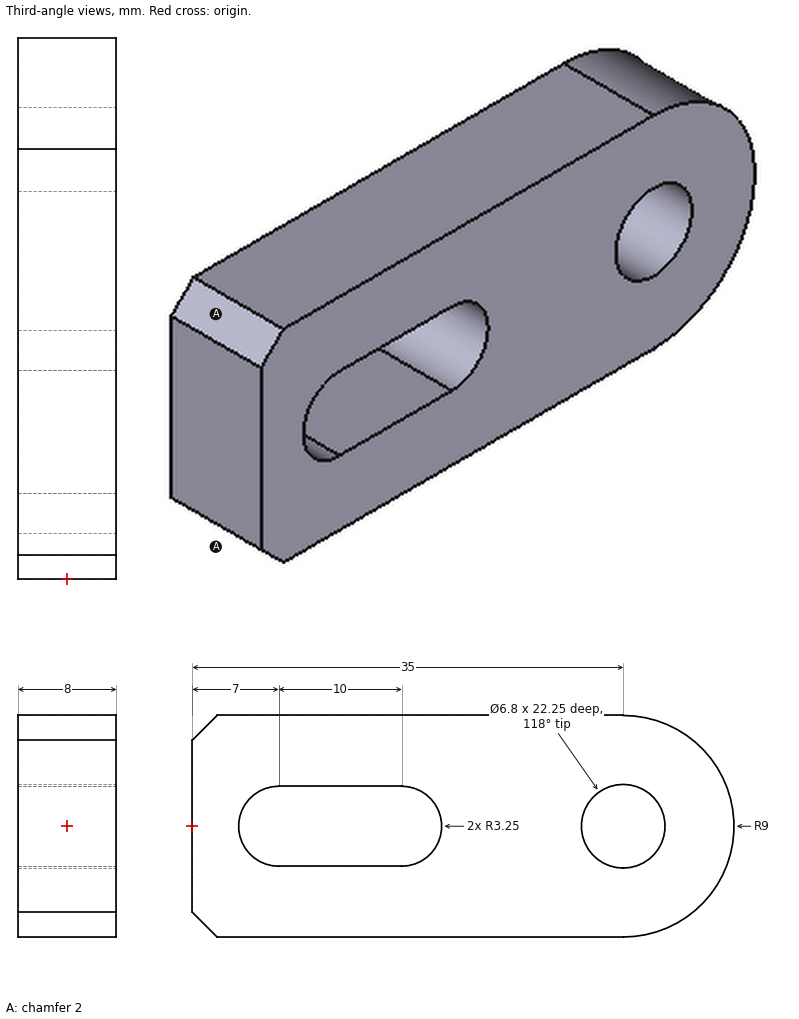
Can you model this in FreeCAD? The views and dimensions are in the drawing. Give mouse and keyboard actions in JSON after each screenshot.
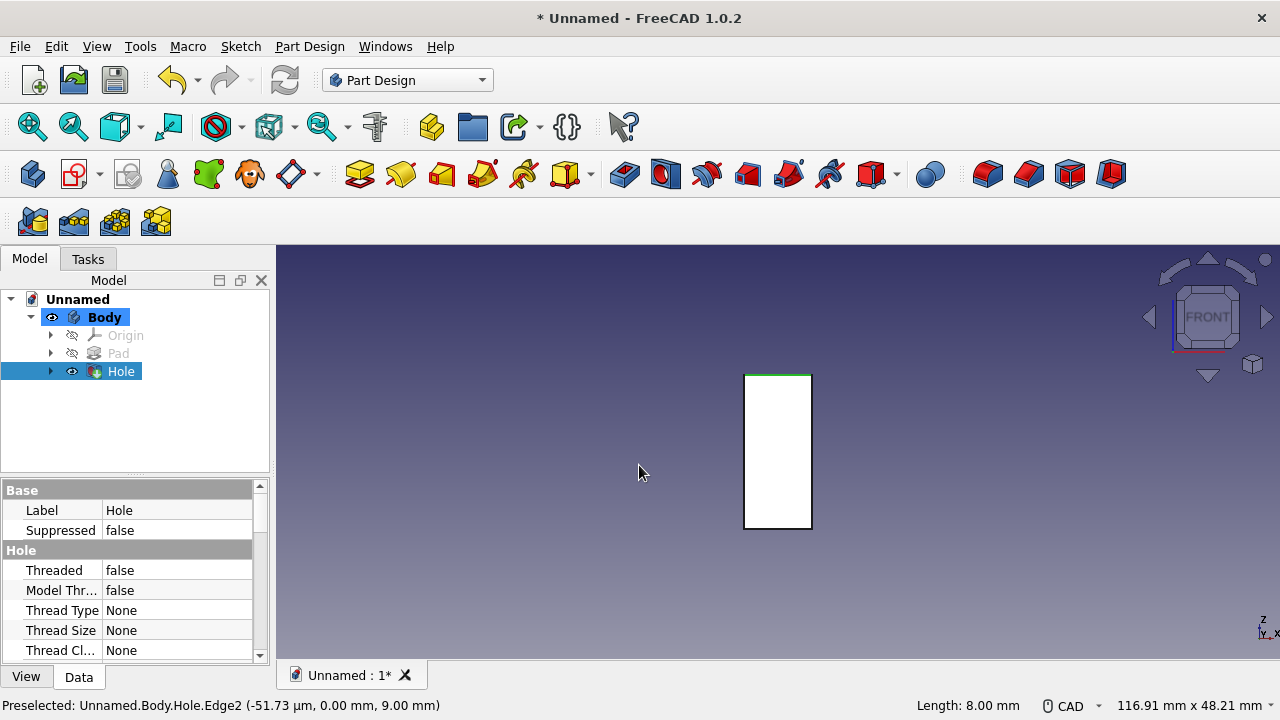
{"action": "key", "text": "v f"}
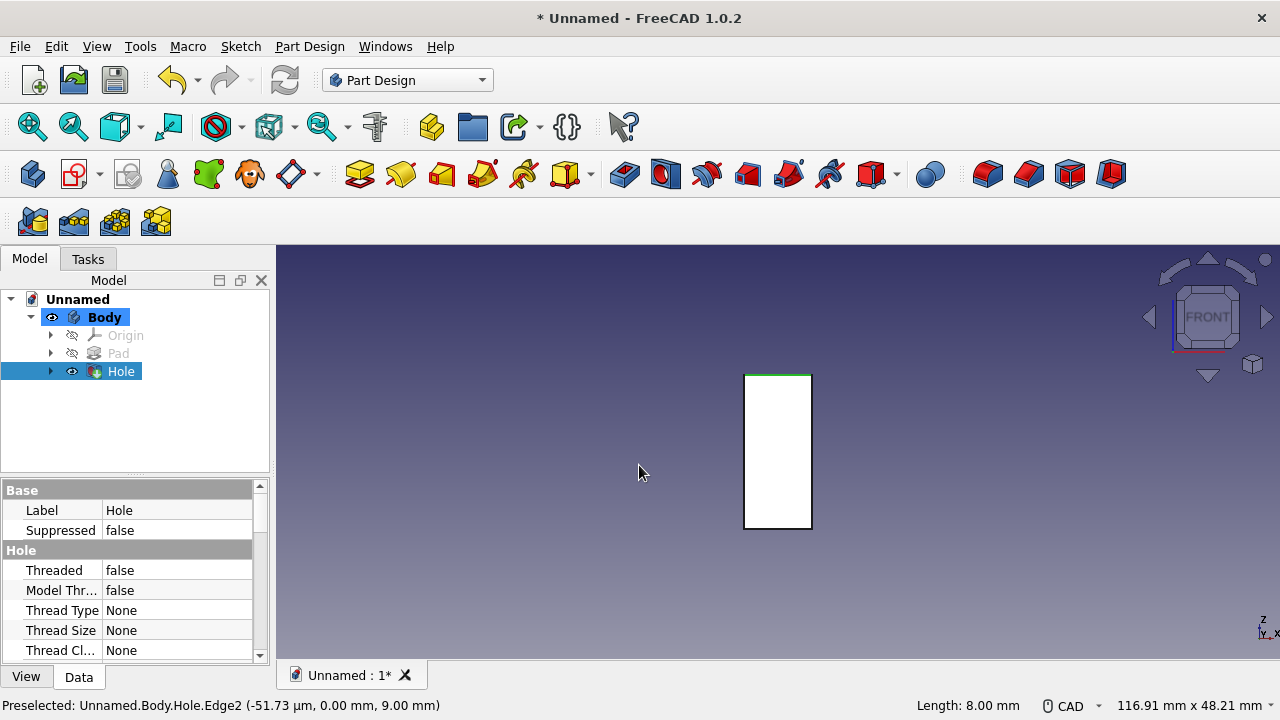
{"action": "left_click", "coordinate": [778, 528], "text": "ctrl"}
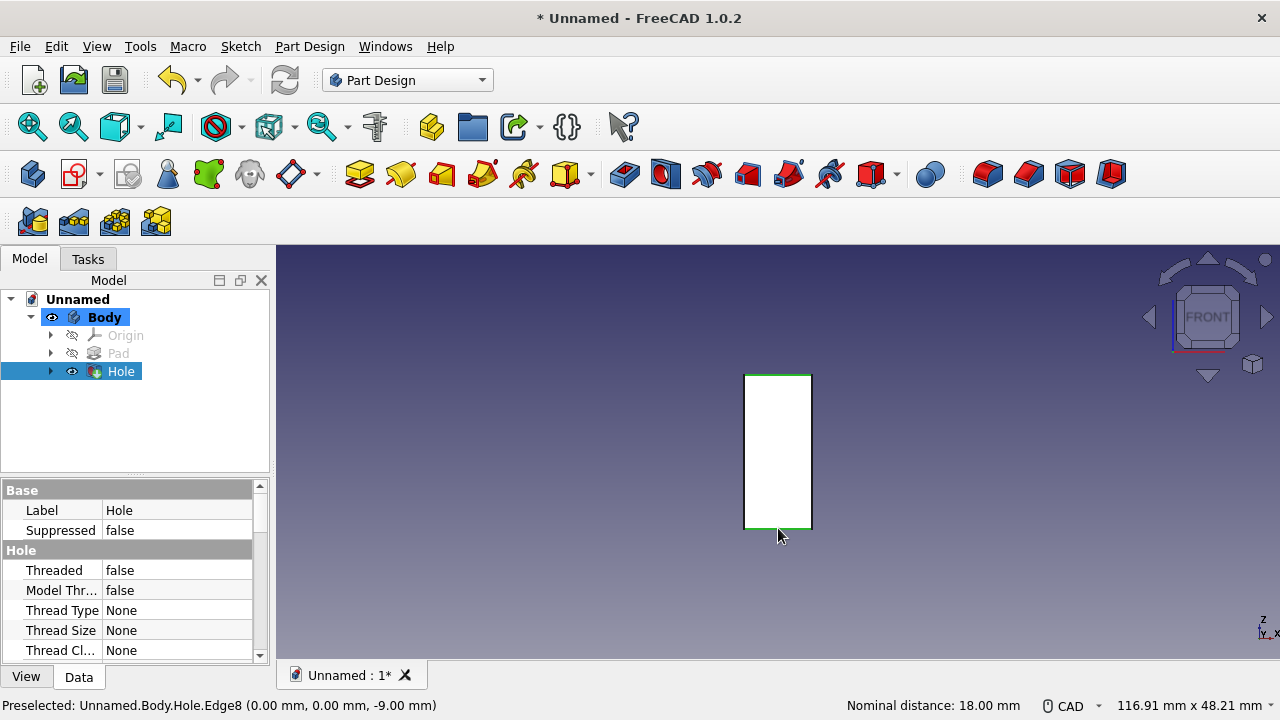
{"action": "left_click", "coordinate": [1029, 174]}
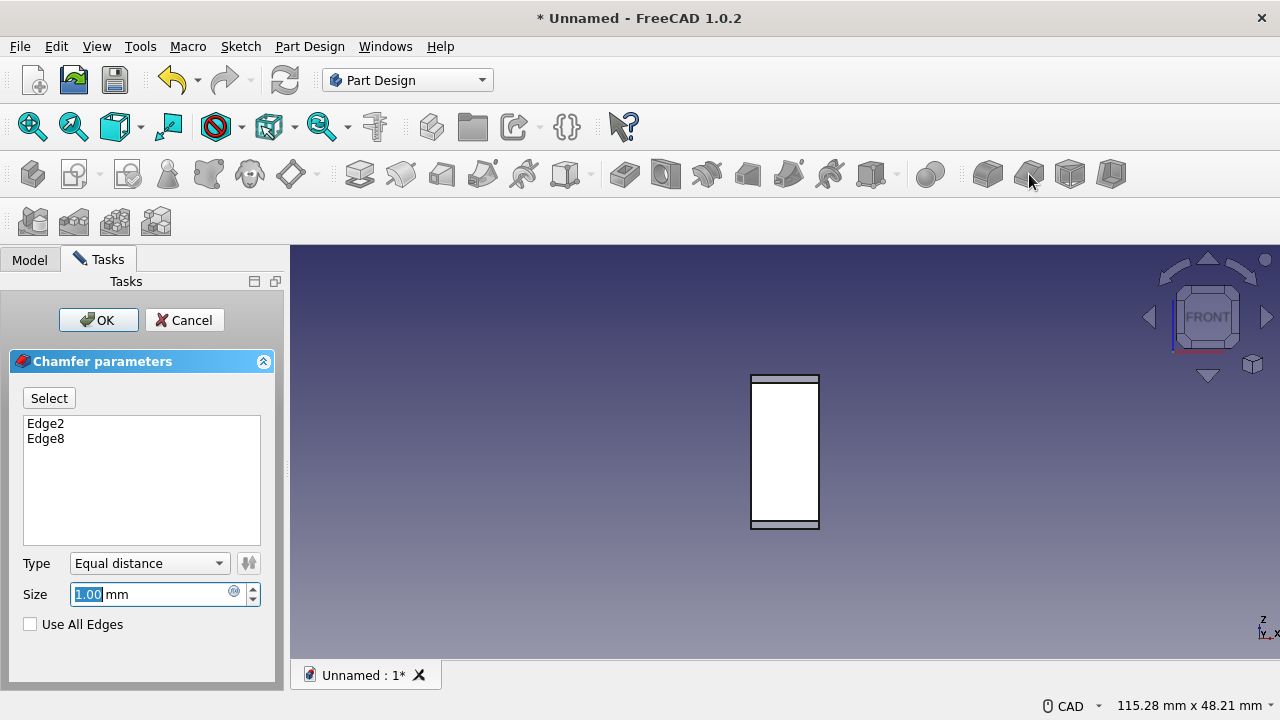
{"action": "type", "text": "2"}
{"action": "key", "text": "Tab"}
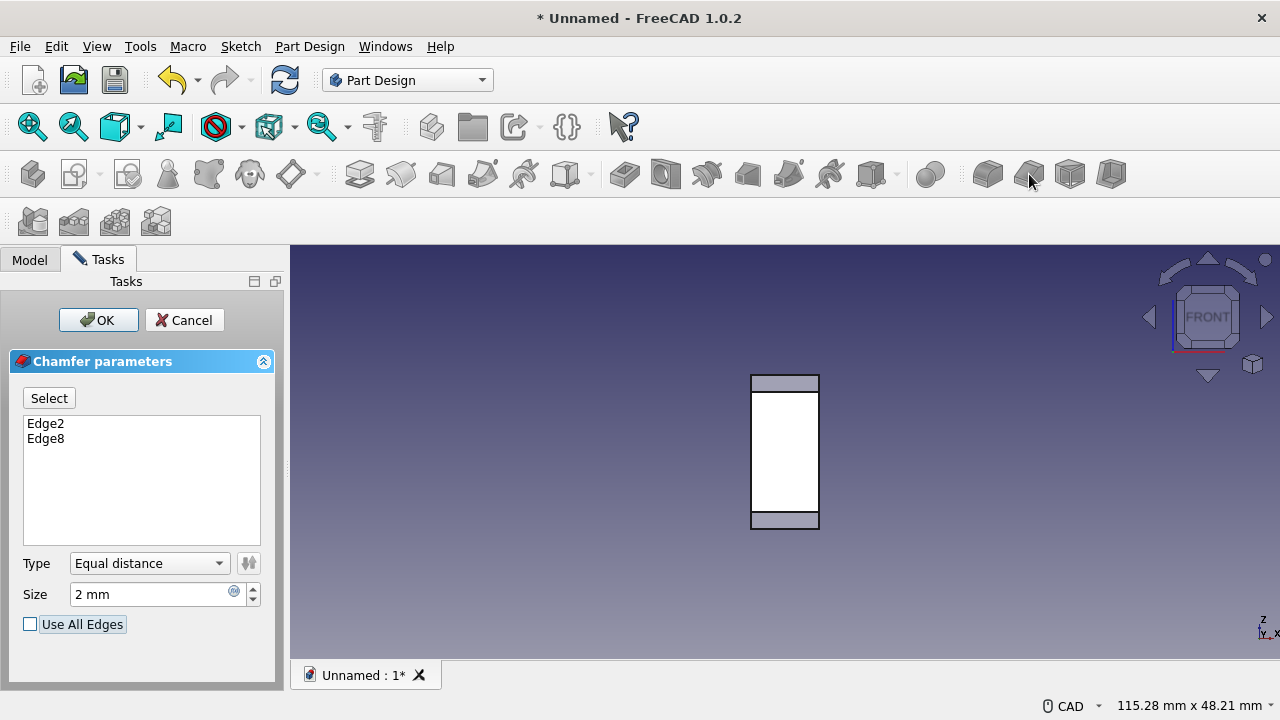
{"action": "left_click", "coordinate": [99, 320]}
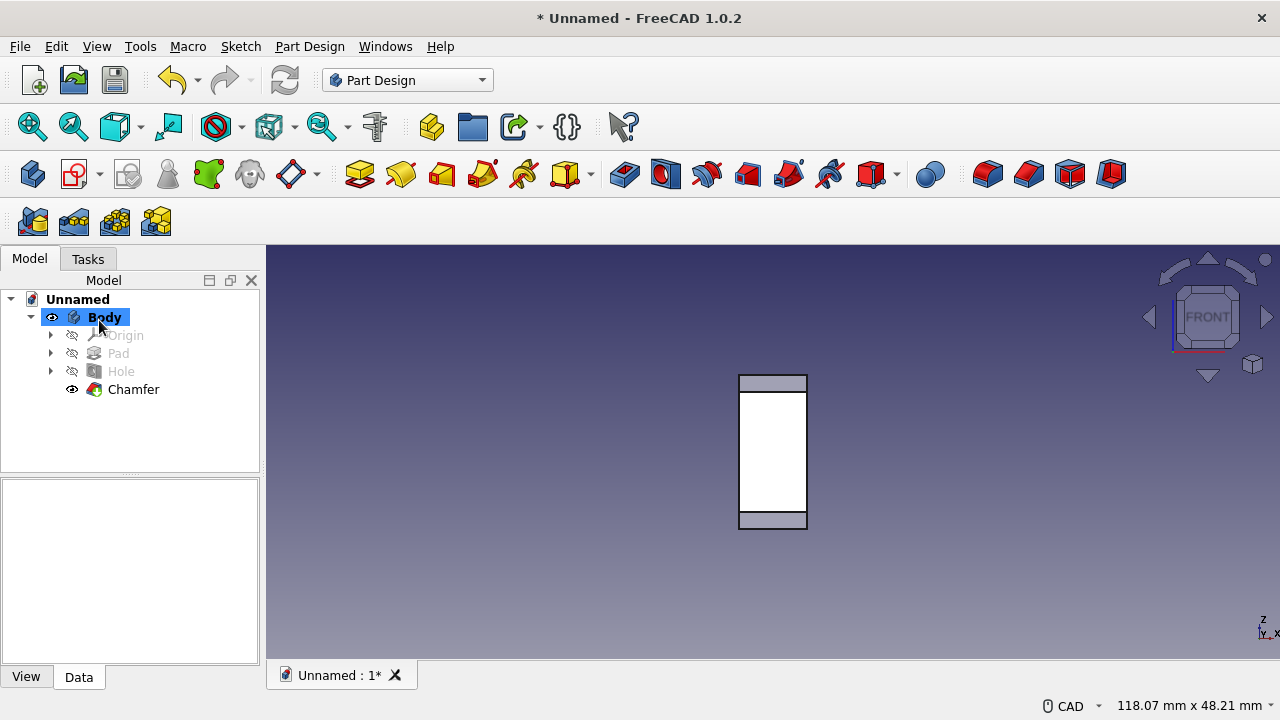
{"action": "key", "text": "0"}